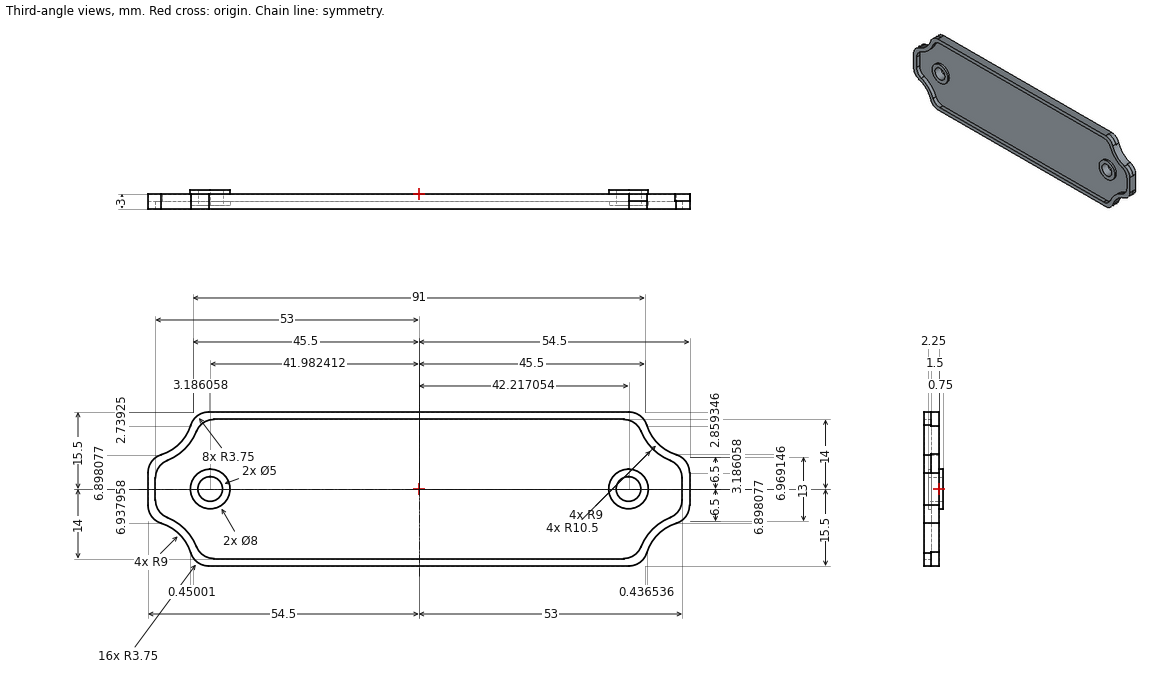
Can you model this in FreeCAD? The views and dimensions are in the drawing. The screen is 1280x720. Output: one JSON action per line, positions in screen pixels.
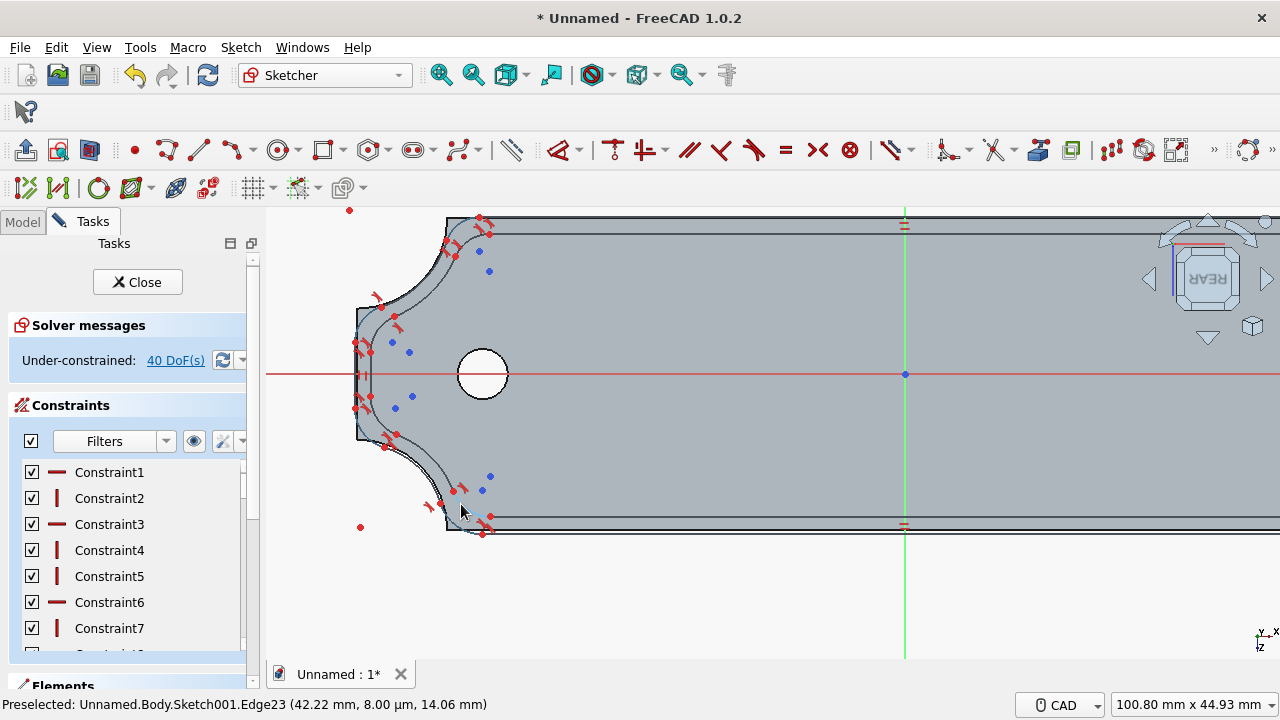
{"action": "left_click", "coordinate": [461, 504]}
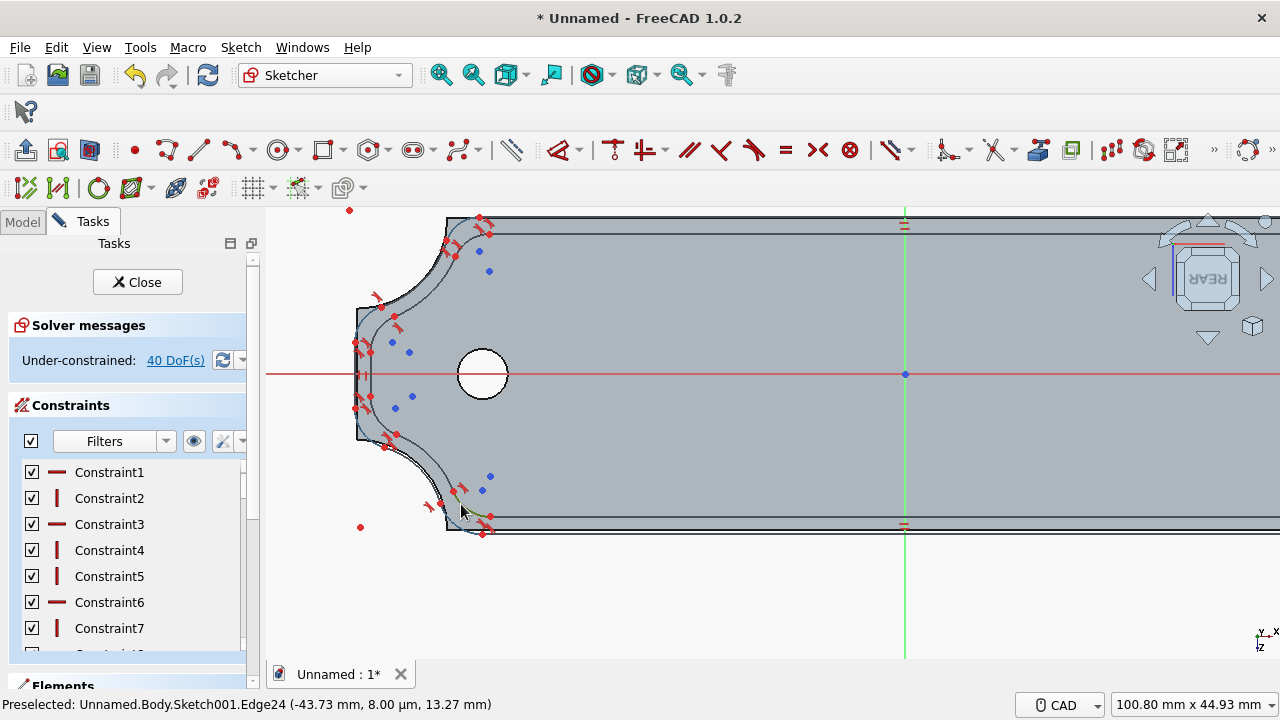
{"action": "left_click", "coordinate": [373, 411]}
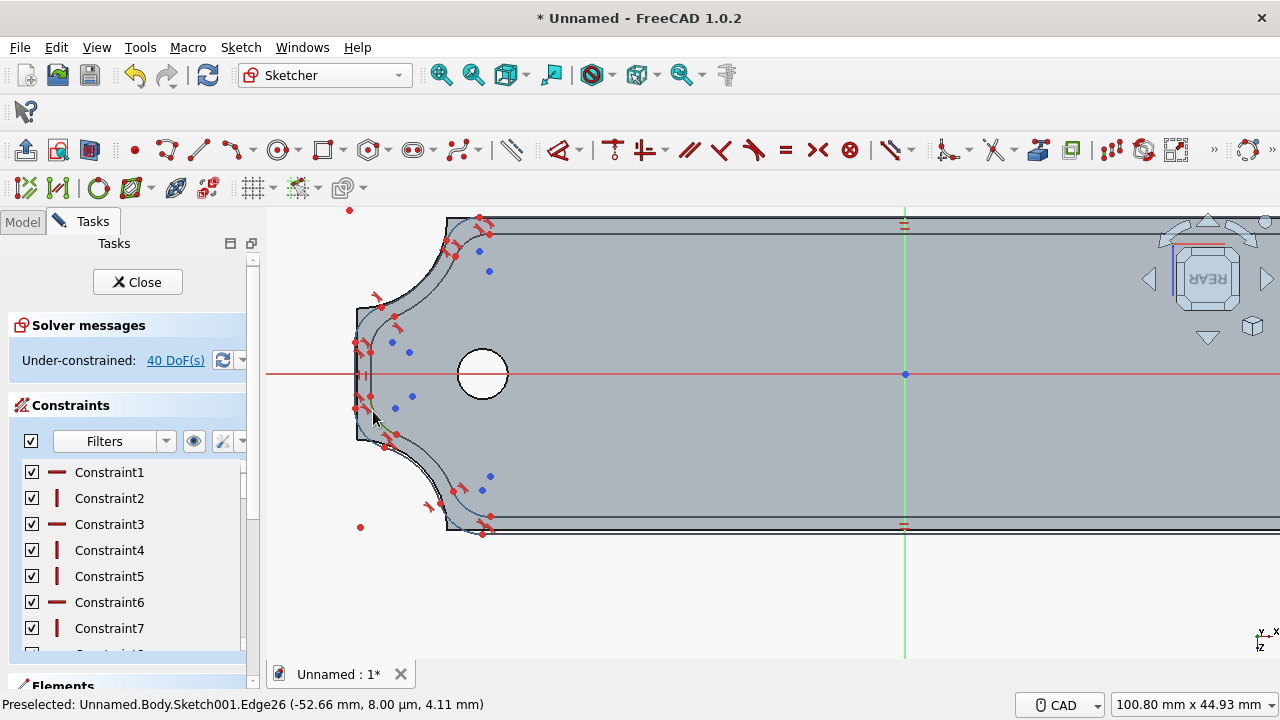
{"action": "left_click", "coordinate": [383, 324]}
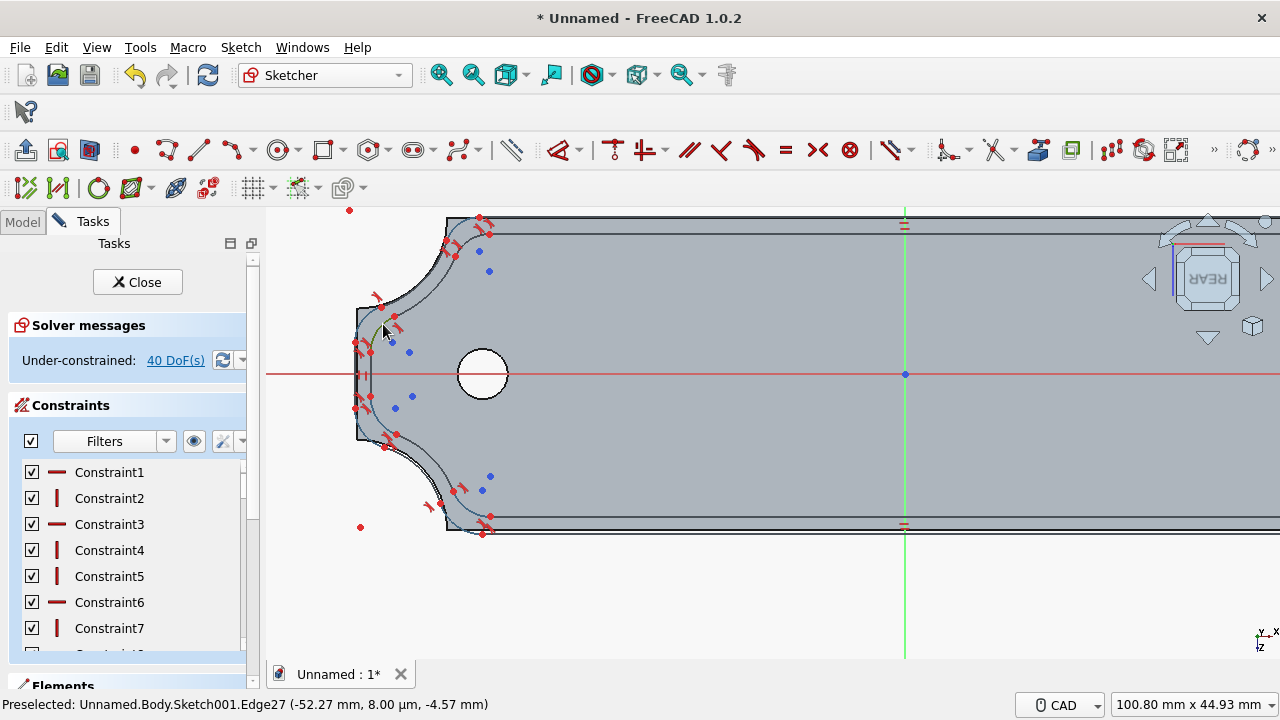
{"action": "left_click", "coordinate": [477, 236]}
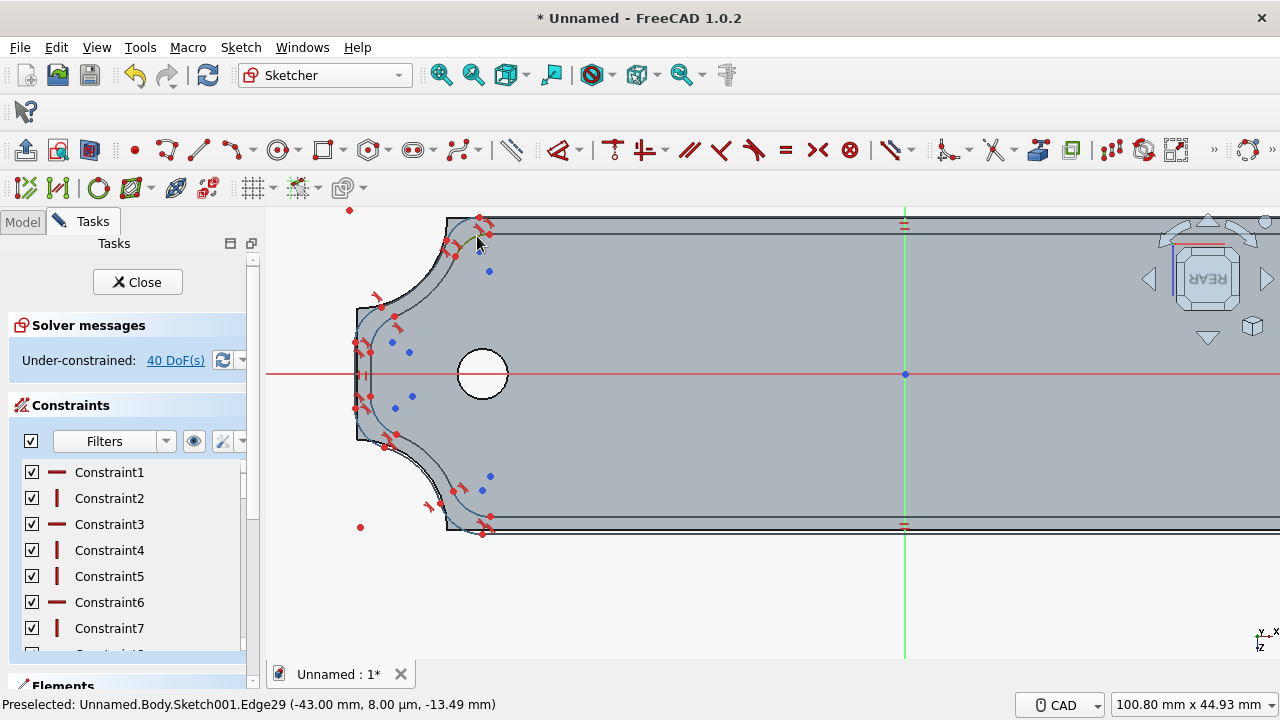
{"action": "scroll", "coordinate": [461, 505], "scroll_direction": "down", "scroll_amount": 3}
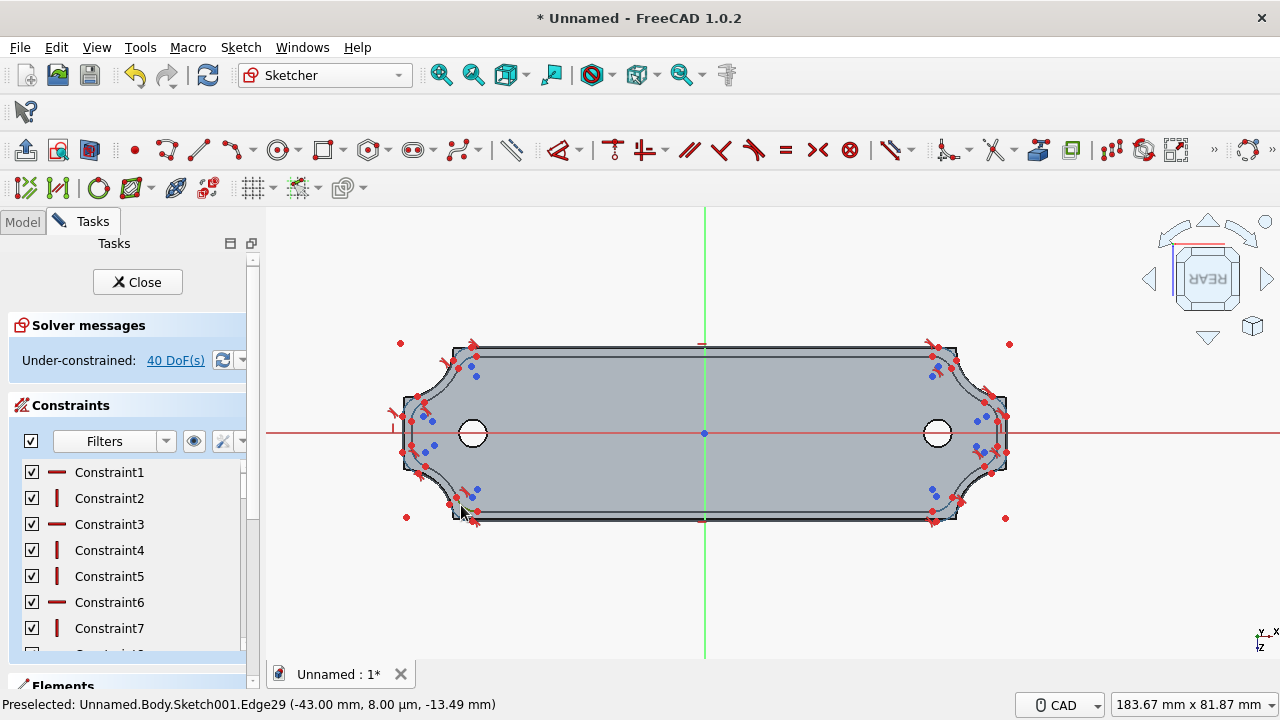
{"action": "scroll", "coordinate": [947, 363], "scroll_direction": "up", "scroll_amount": 4}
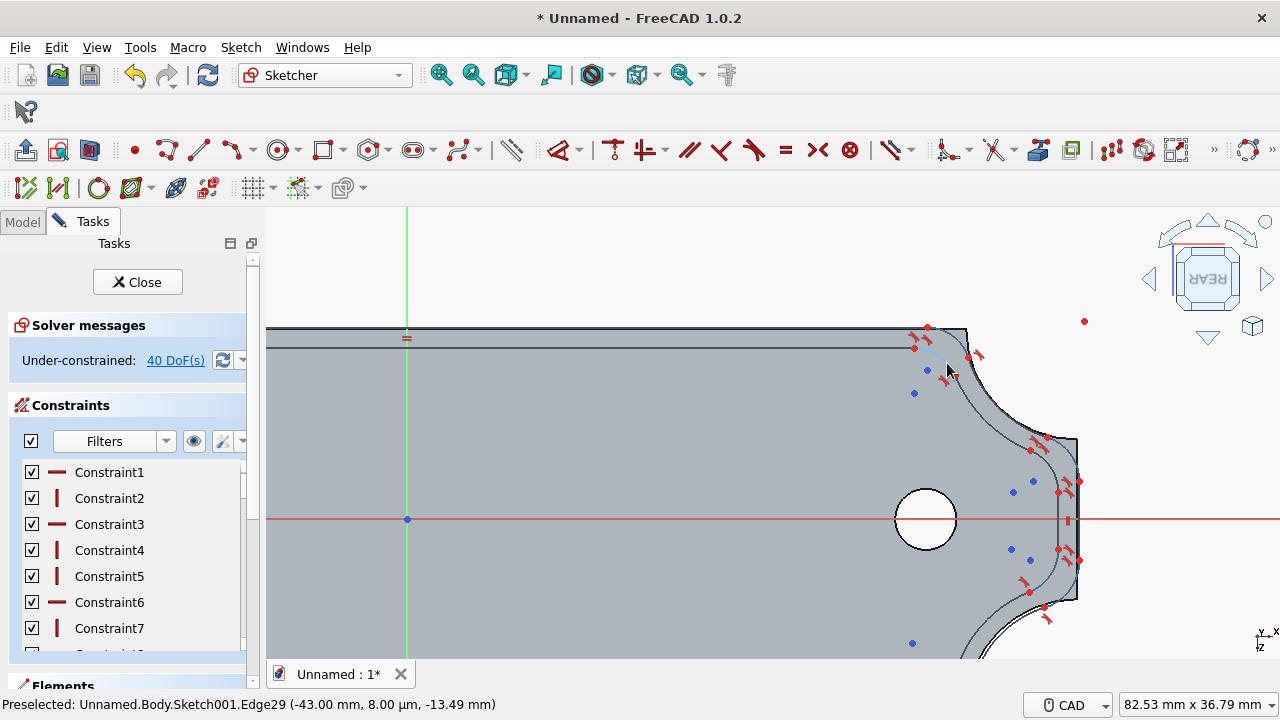
{"action": "left_click", "coordinate": [947, 363]}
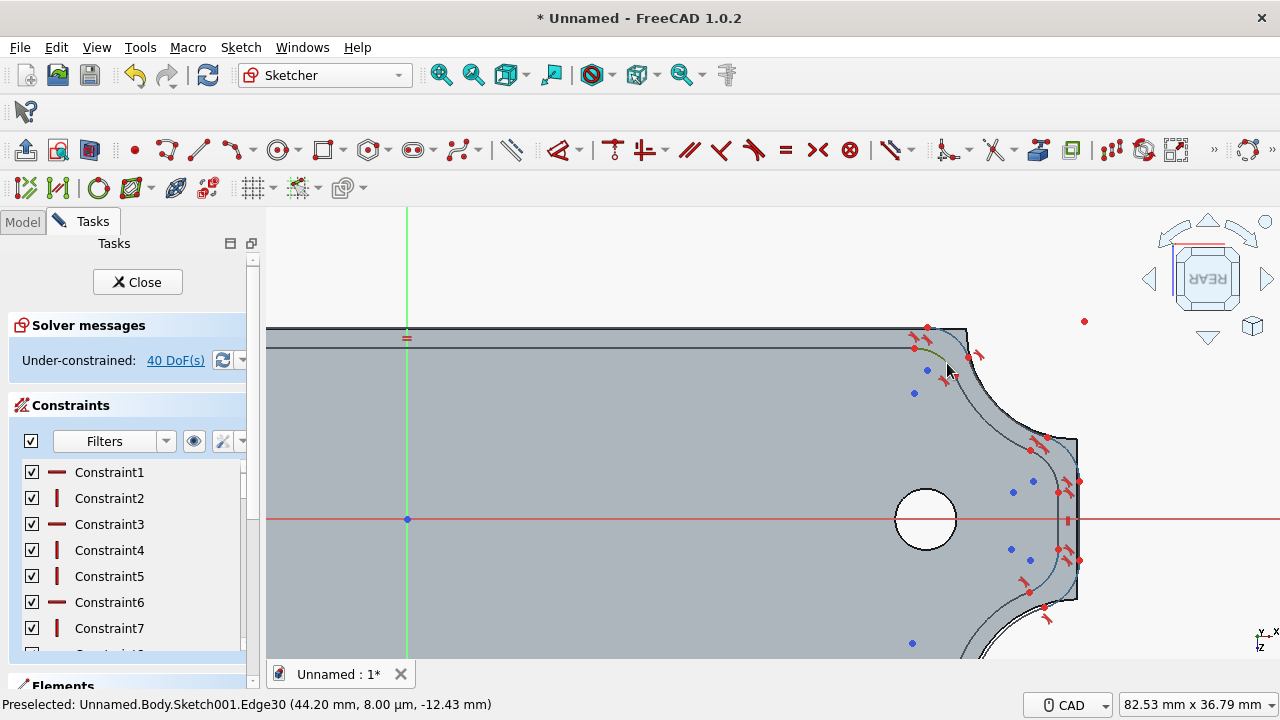
{"action": "left_click", "coordinate": [1056, 477]}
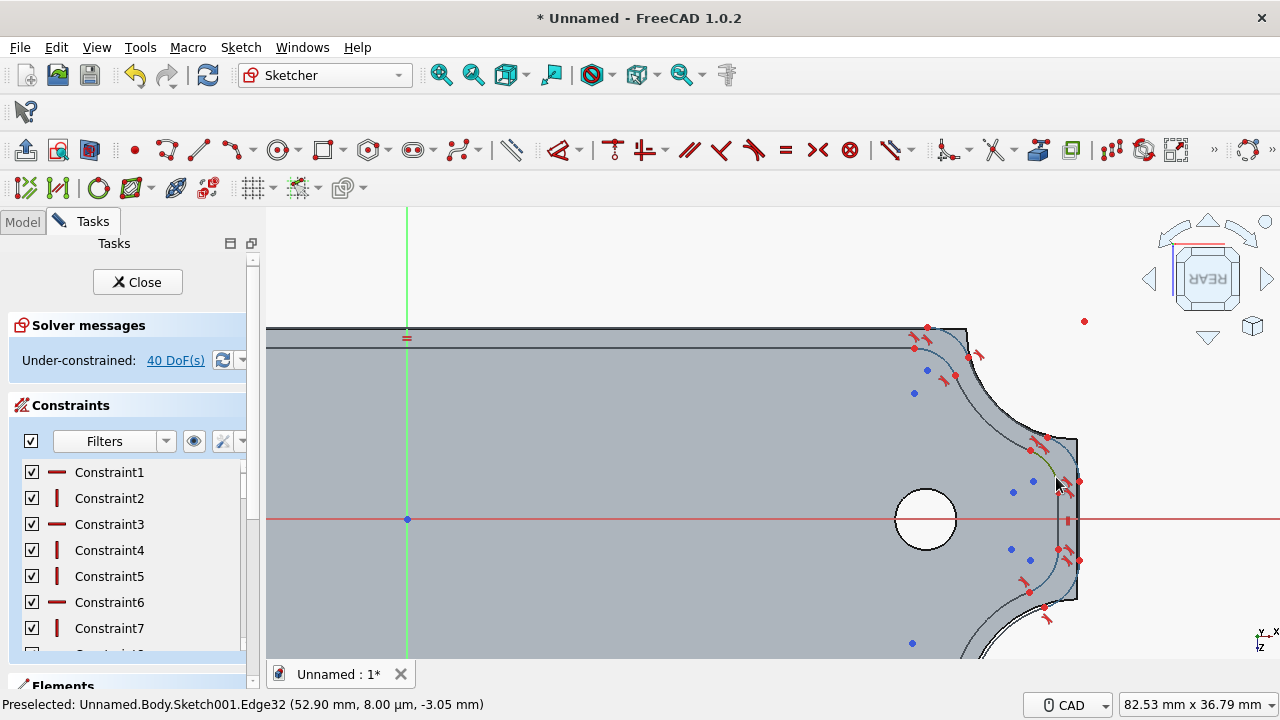
{"action": "left_click", "coordinate": [786, 150]}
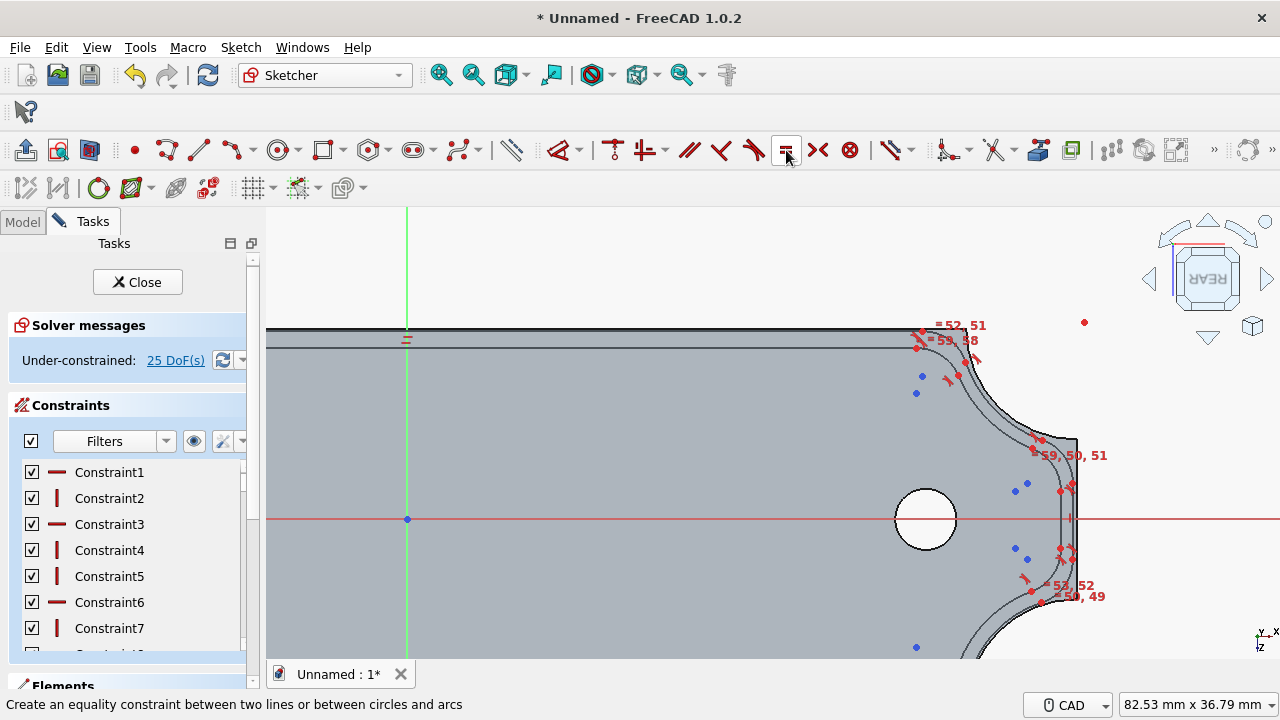
{"action": "scroll", "coordinate": [947, 363], "scroll_direction": "down", "scroll_amount": 4}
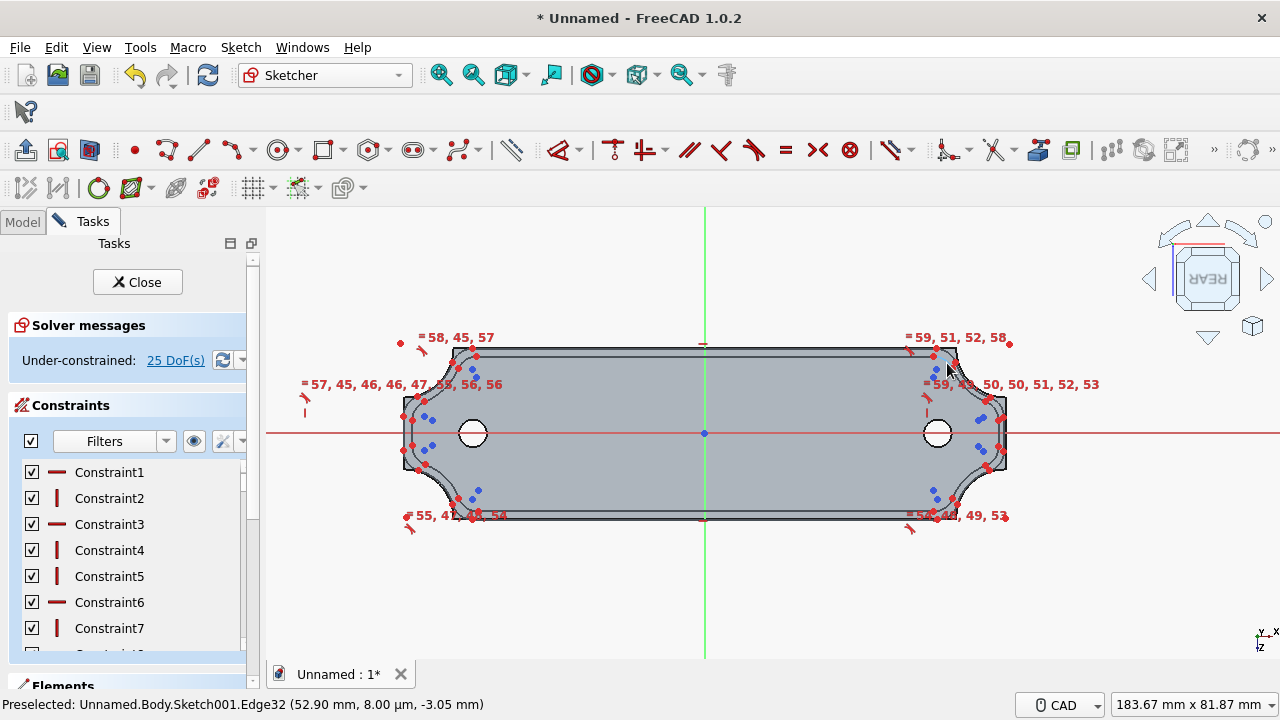
{"action": "scroll", "coordinate": [431, 390], "scroll_direction": "up", "scroll_amount": 4}